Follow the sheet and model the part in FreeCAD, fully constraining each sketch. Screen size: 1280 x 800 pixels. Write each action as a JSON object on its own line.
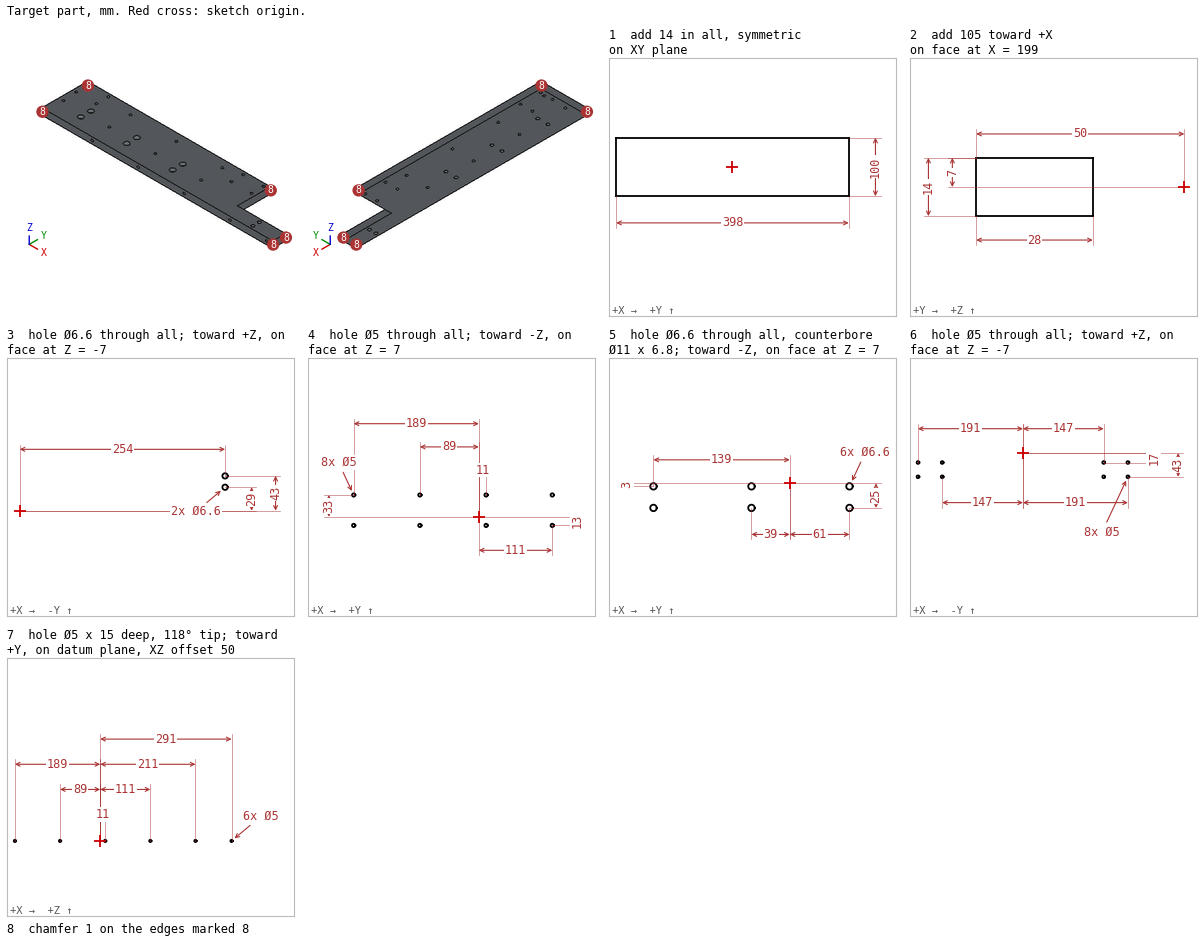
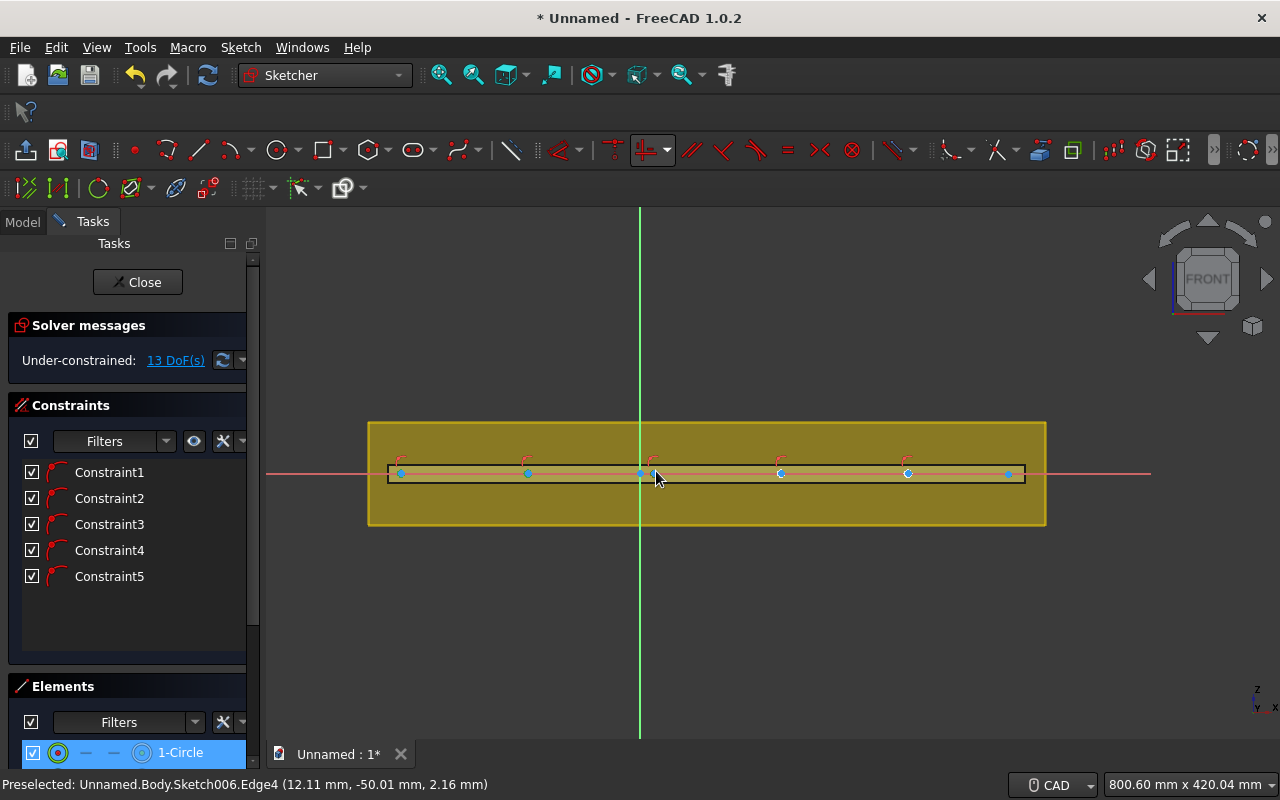
{"action": "scroll", "coordinate": [783, 471], "scroll_direction": "up", "scroll_amount": 9}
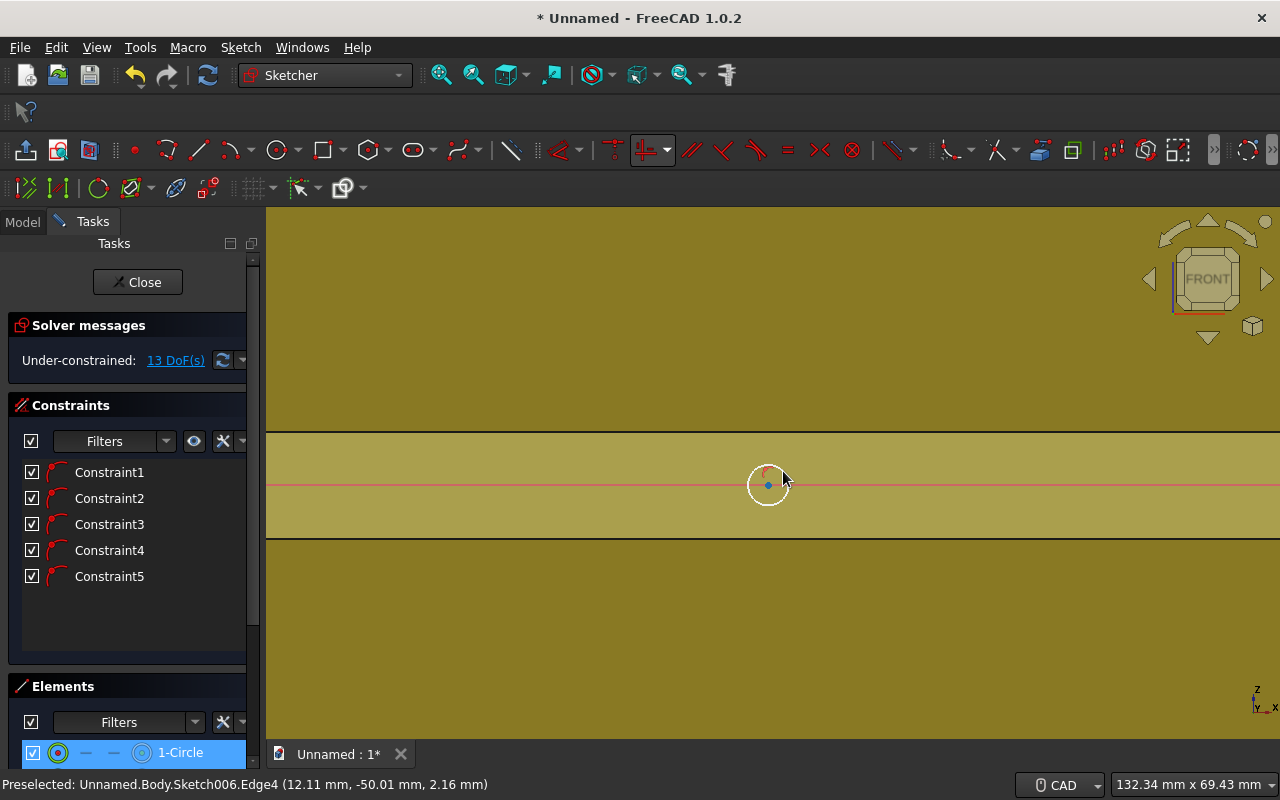
{"action": "left_click", "coordinate": [783, 471]}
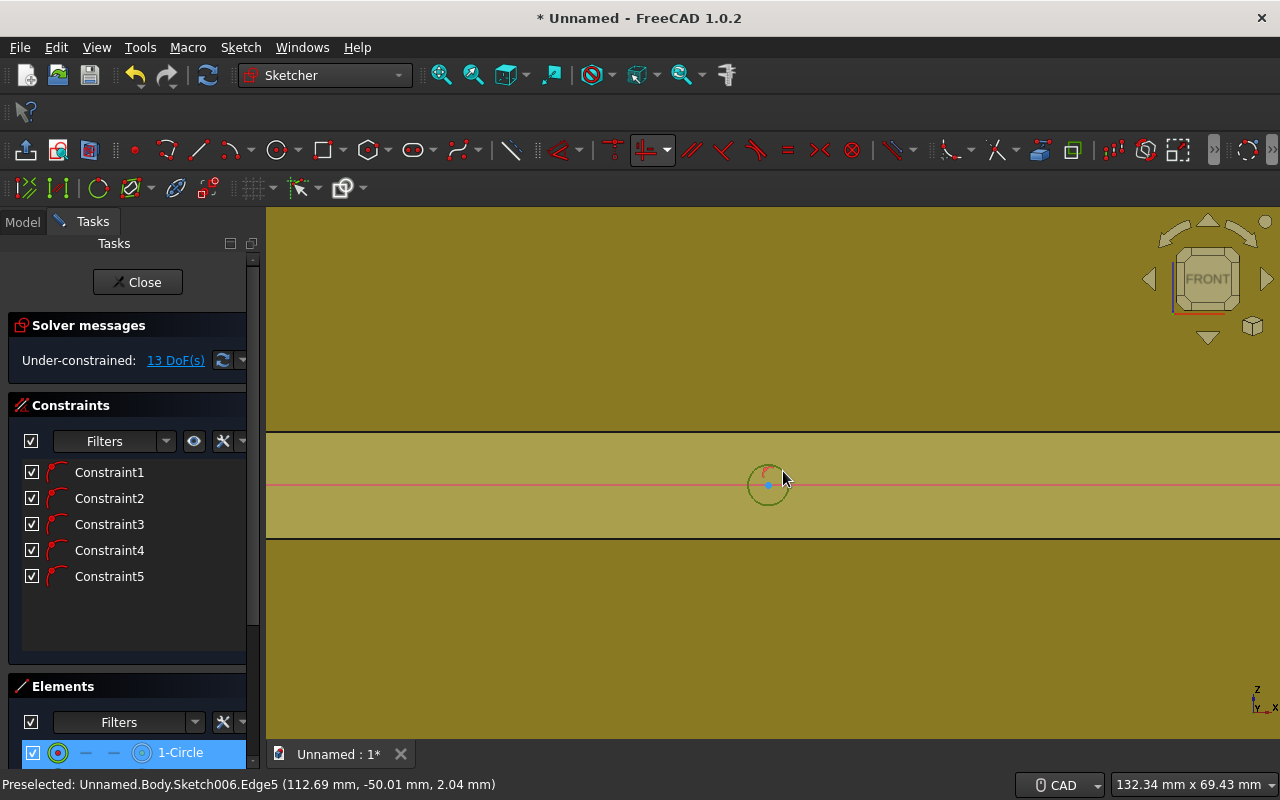
{"action": "scroll", "coordinate": [783, 471], "scroll_direction": "down", "scroll_amount": 9}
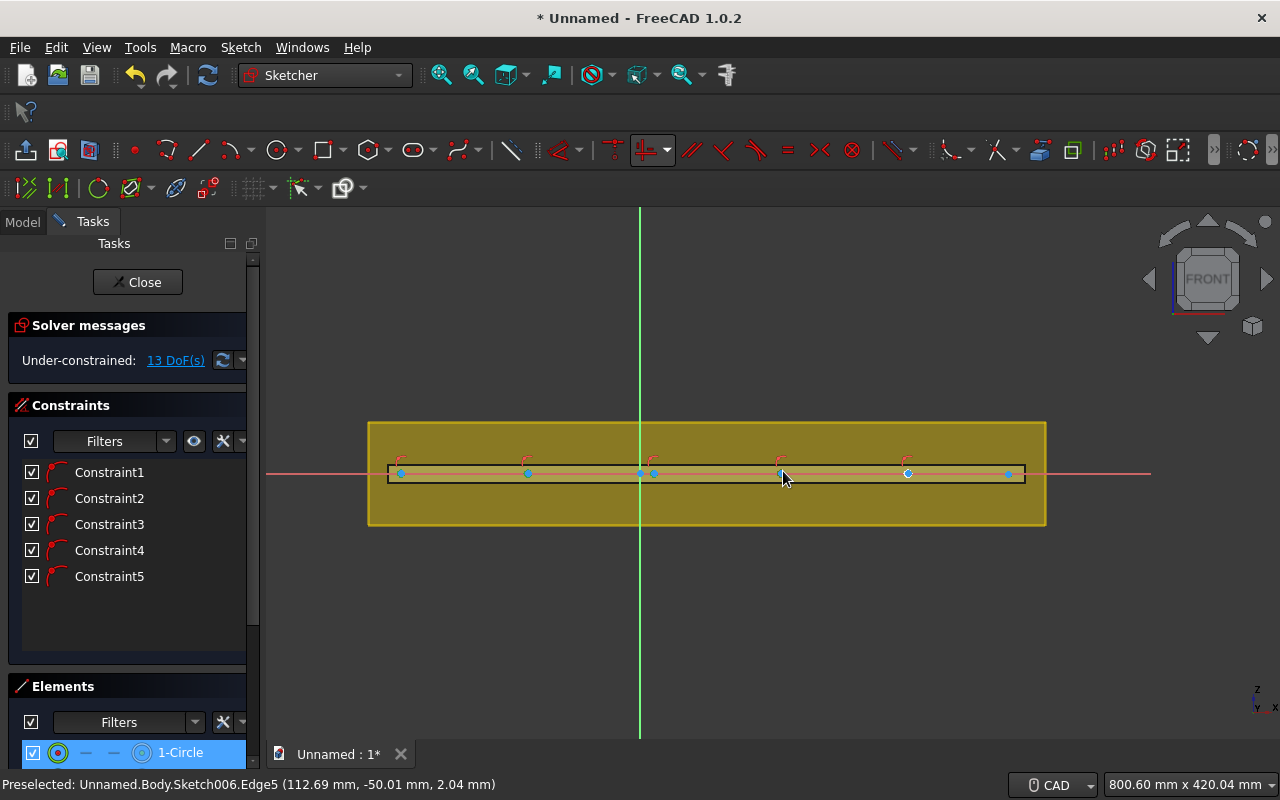
{"action": "scroll", "coordinate": [910, 471], "scroll_direction": "up", "scroll_amount": 9}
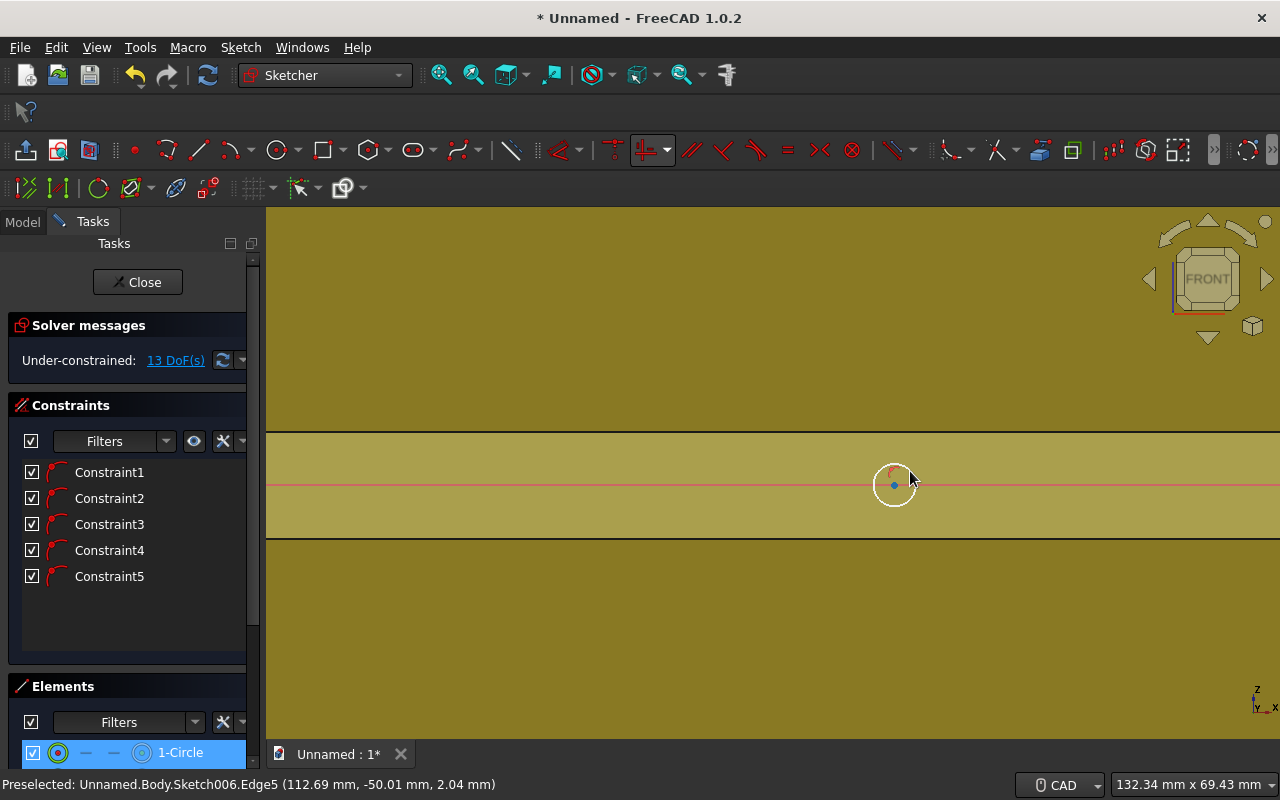
{"action": "left_click", "coordinate": [910, 470]}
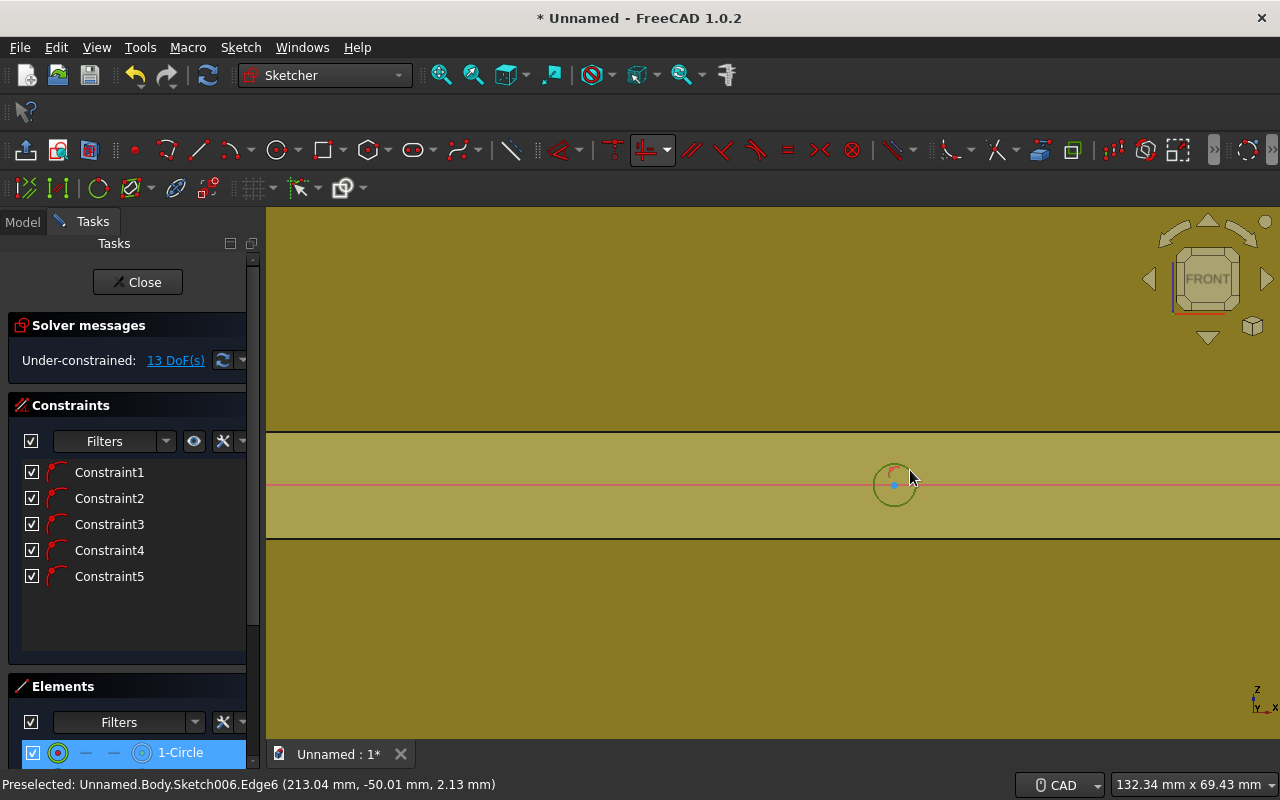
{"action": "key", "text": "e"}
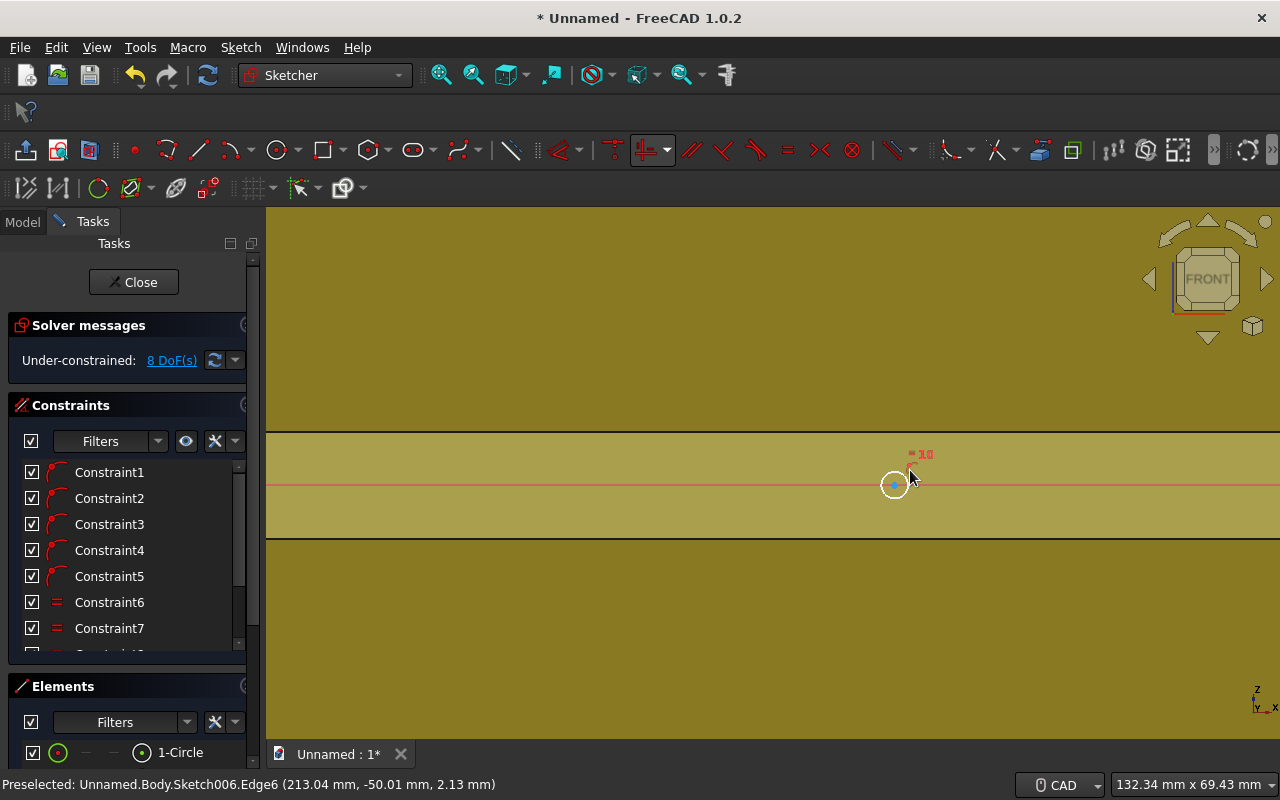
{"action": "scroll", "coordinate": [910, 471], "scroll_direction": "down", "scroll_amount": 9}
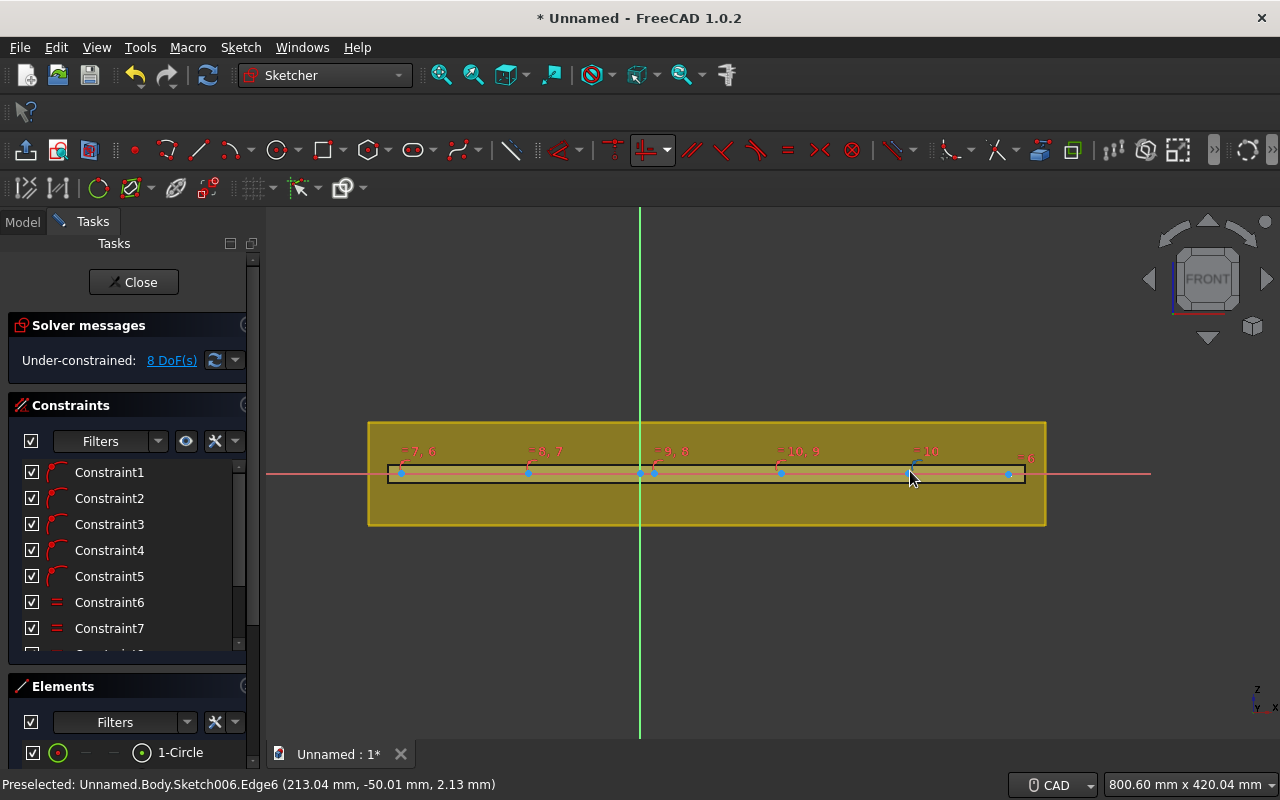
{"action": "left_click", "coordinate": [1009, 475]}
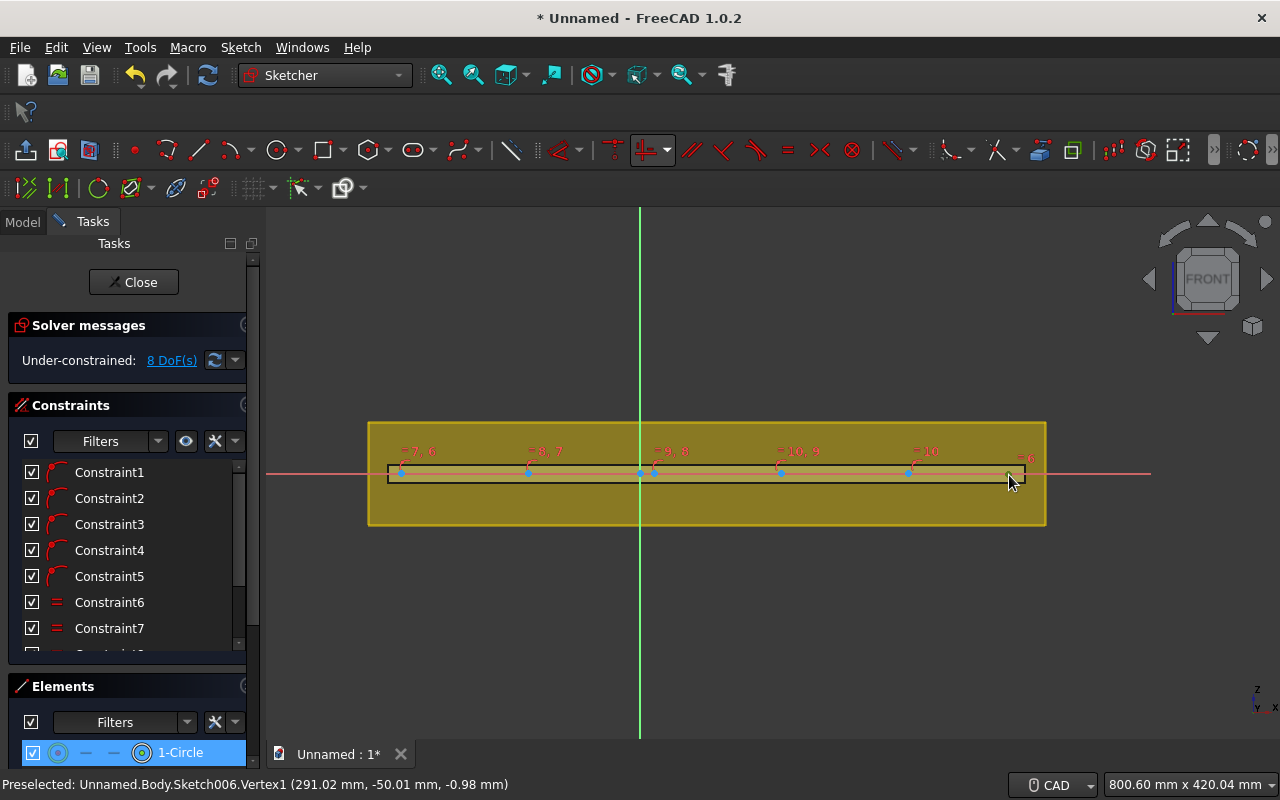
{"action": "left_click", "coordinate": [353, 474]}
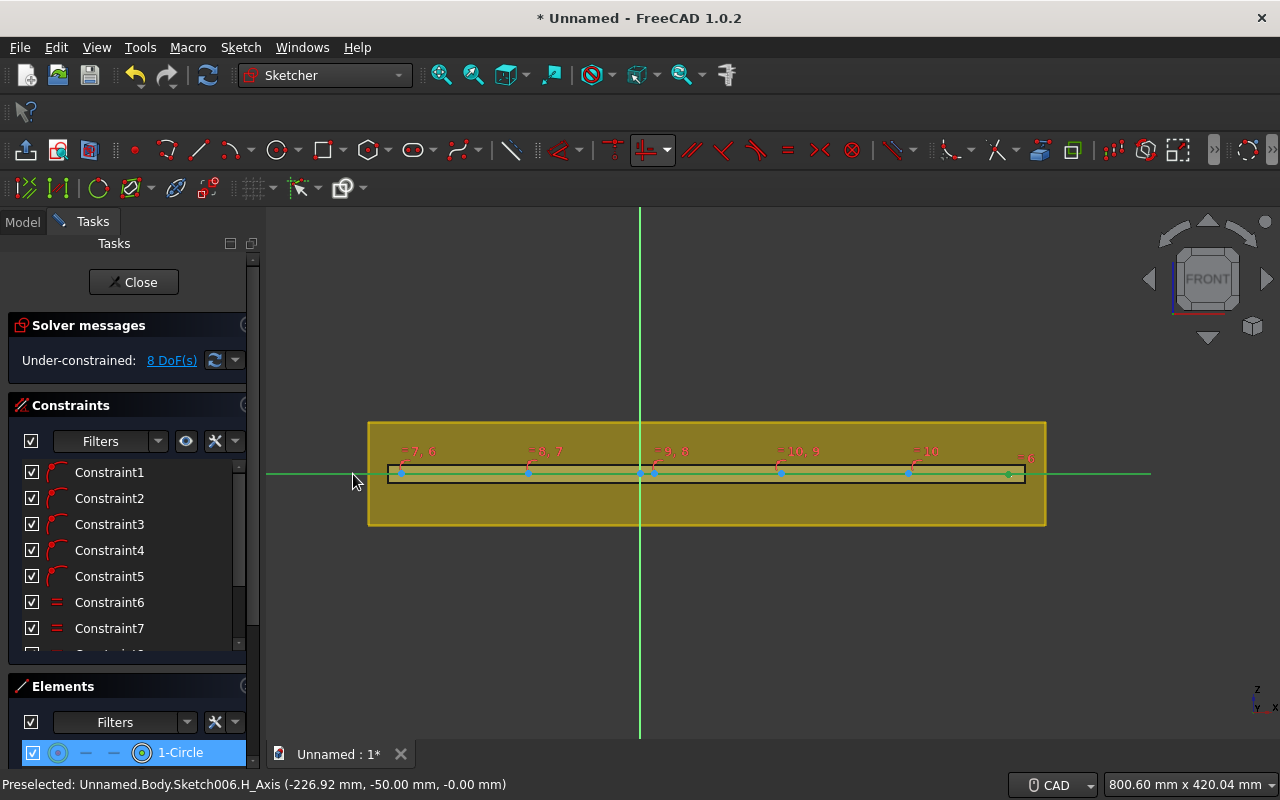
{"action": "key", "text": "c"}